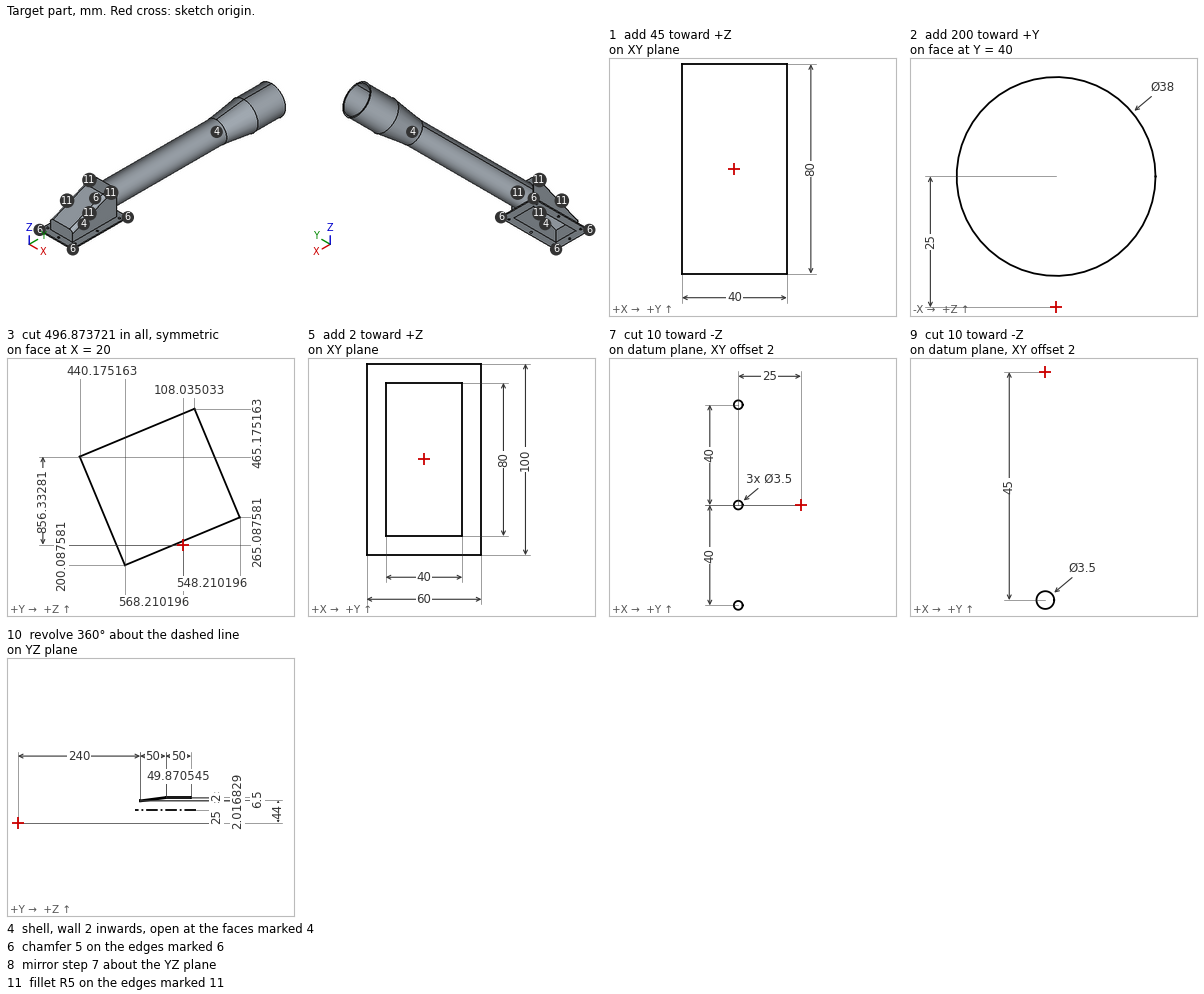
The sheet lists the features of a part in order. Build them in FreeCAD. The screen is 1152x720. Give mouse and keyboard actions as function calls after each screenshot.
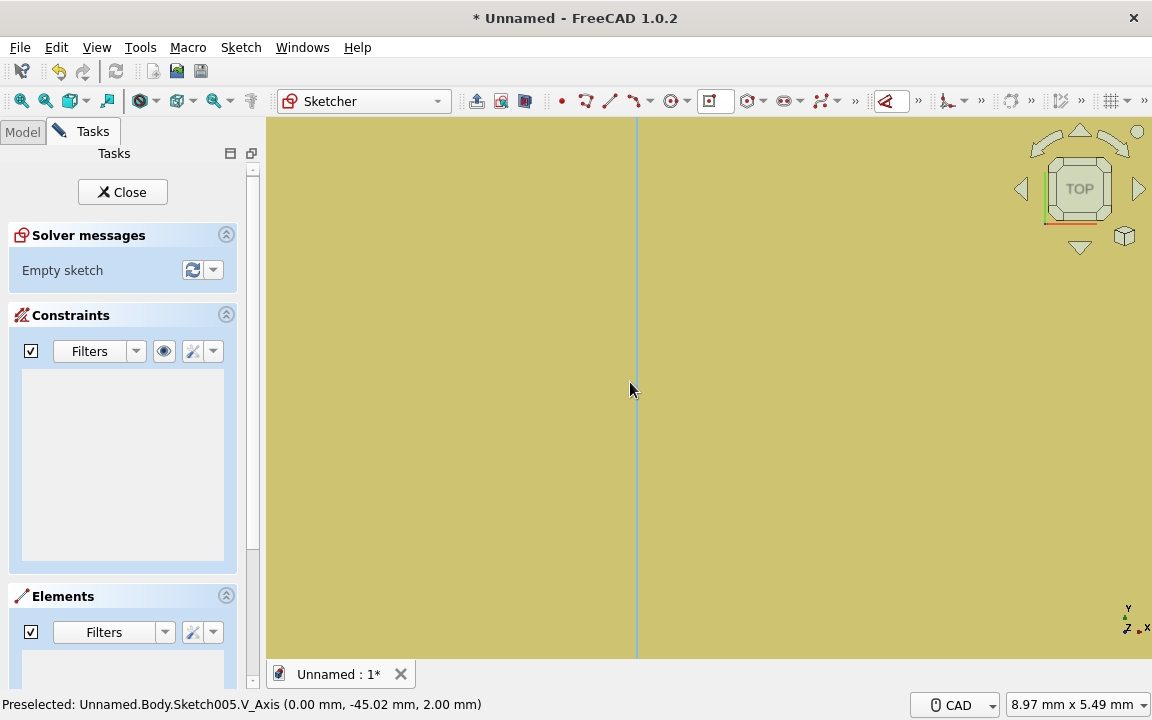
click(672, 102)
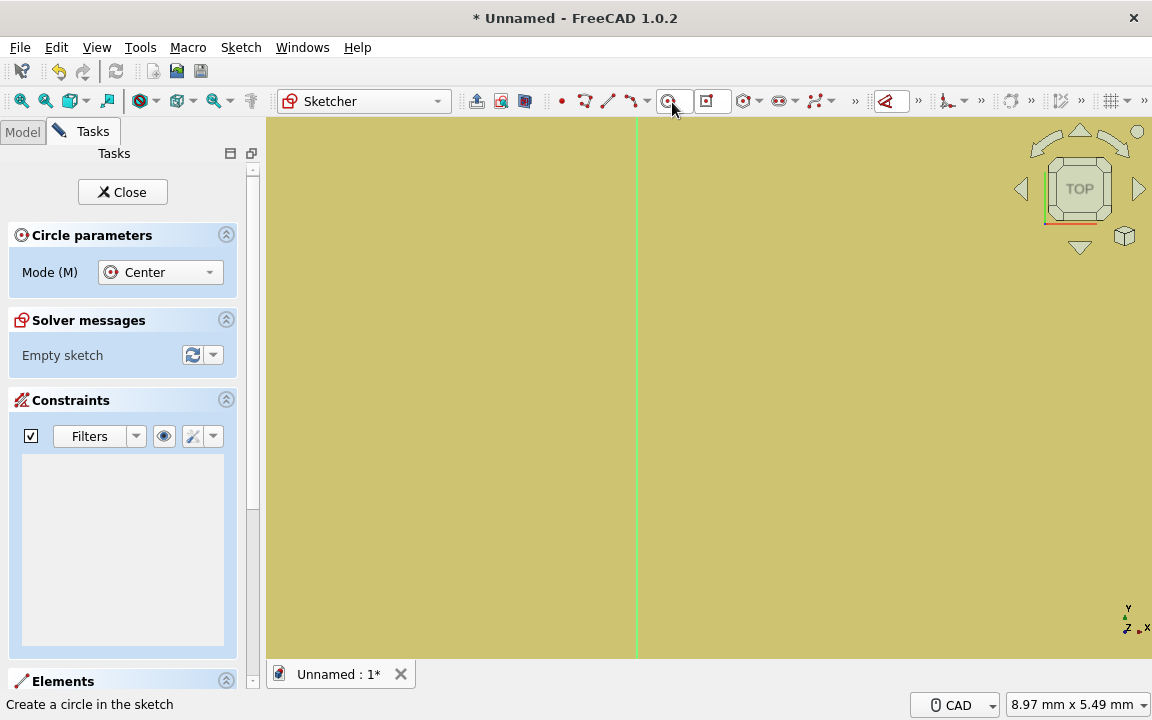
click(637, 384)
move(759, 262)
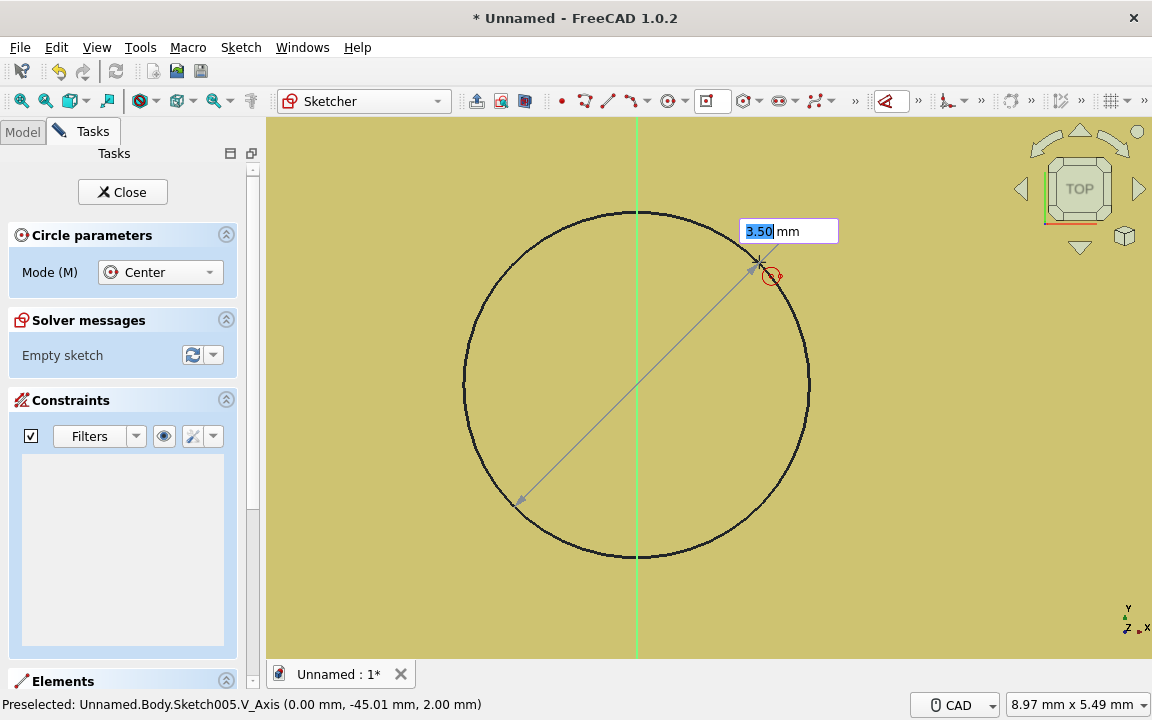
text(3.5)
key(Return)
key(Escape)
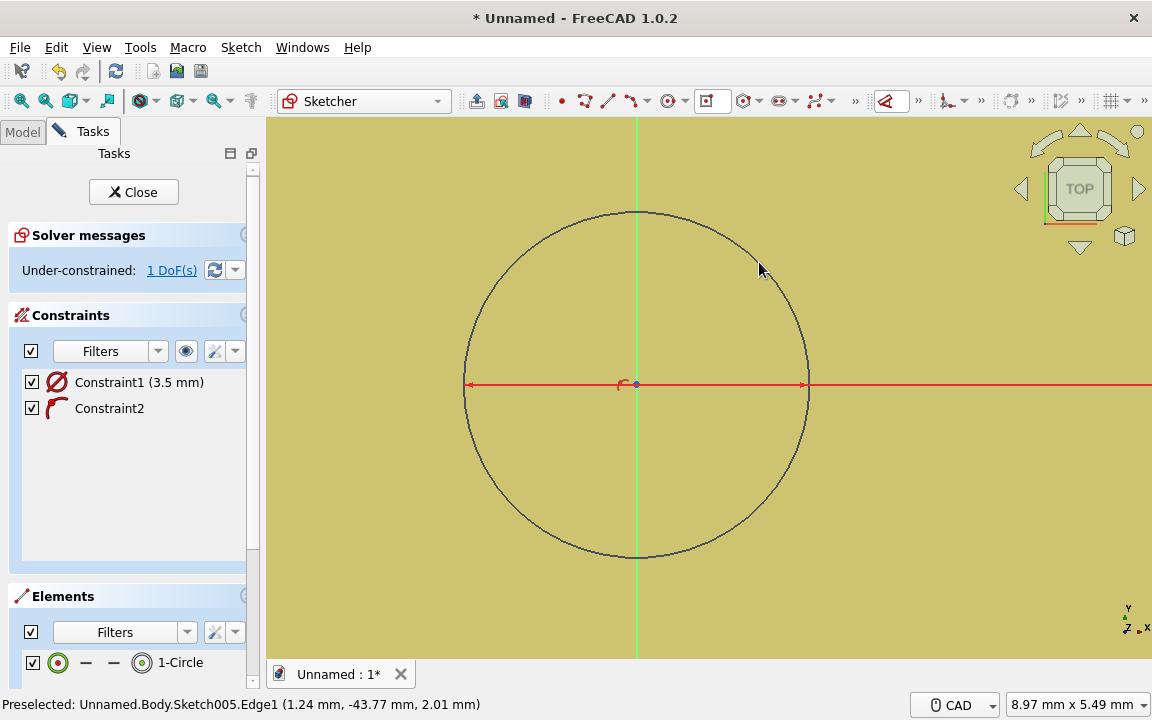
click(886, 102)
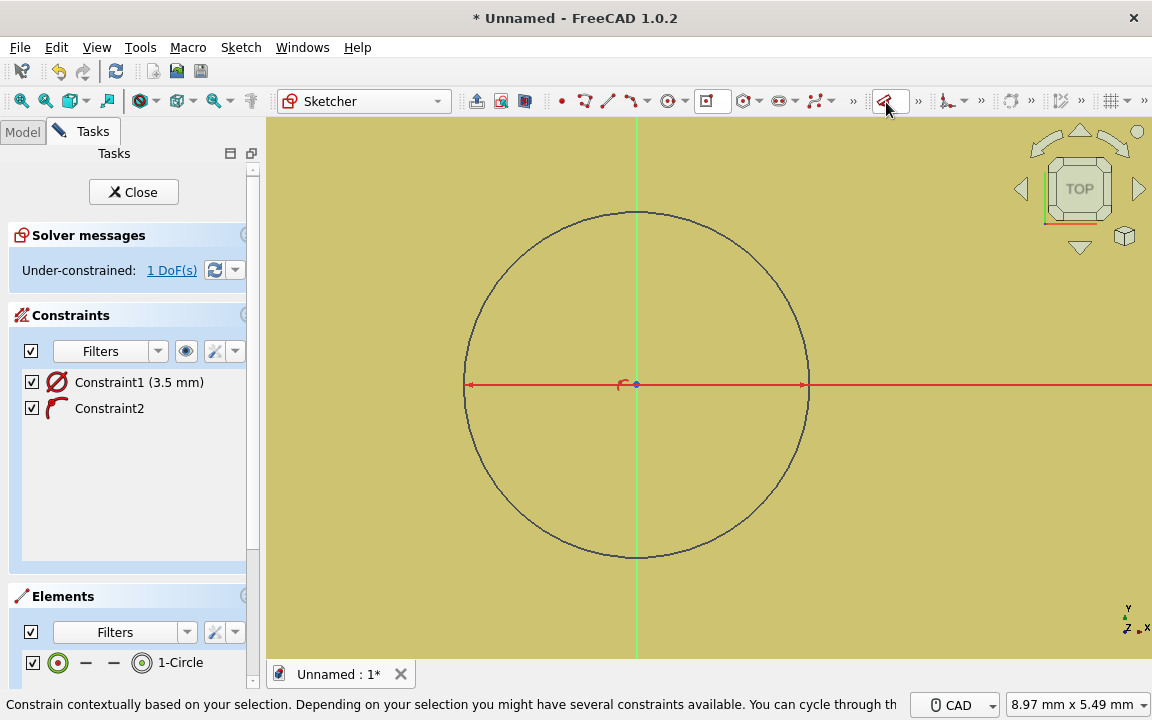
click(637, 385)
click(671, 265)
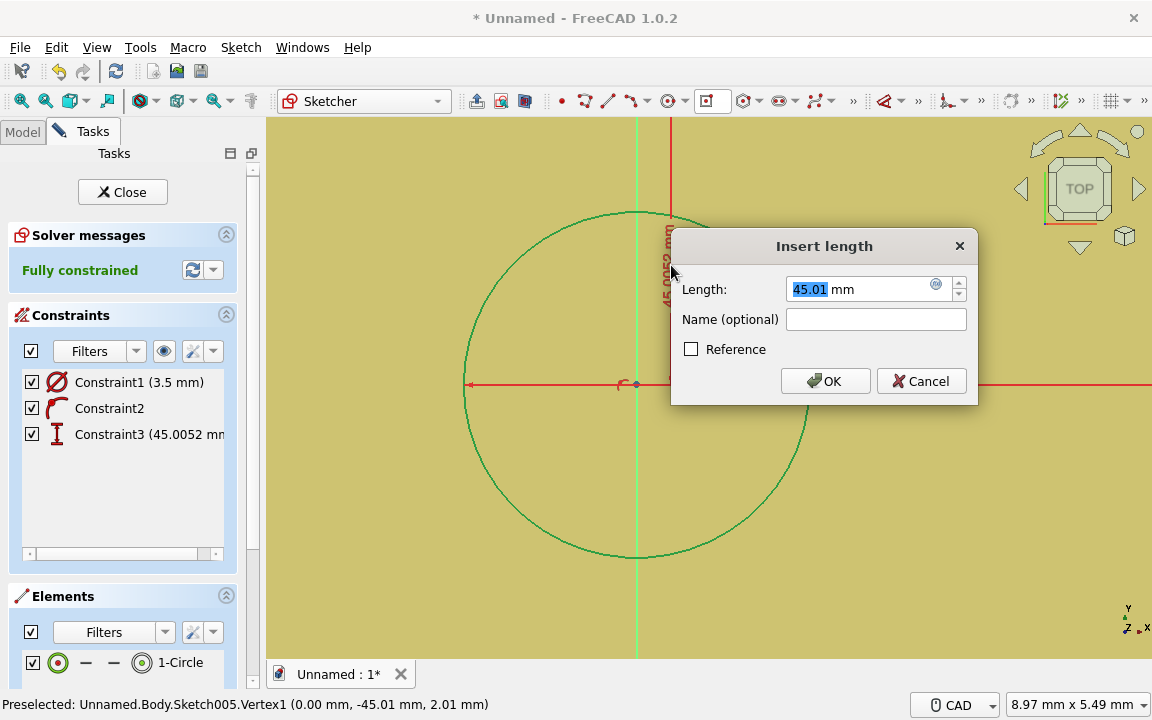
text(45)
key(Return)
key(Escape)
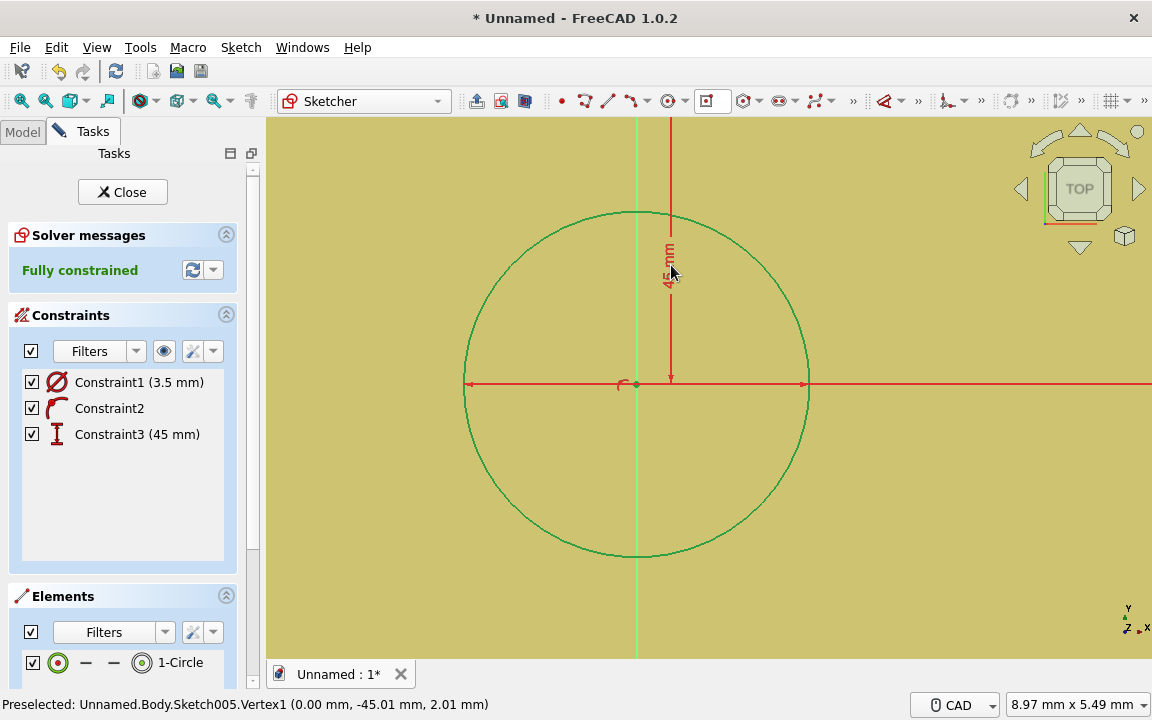
click(123, 192)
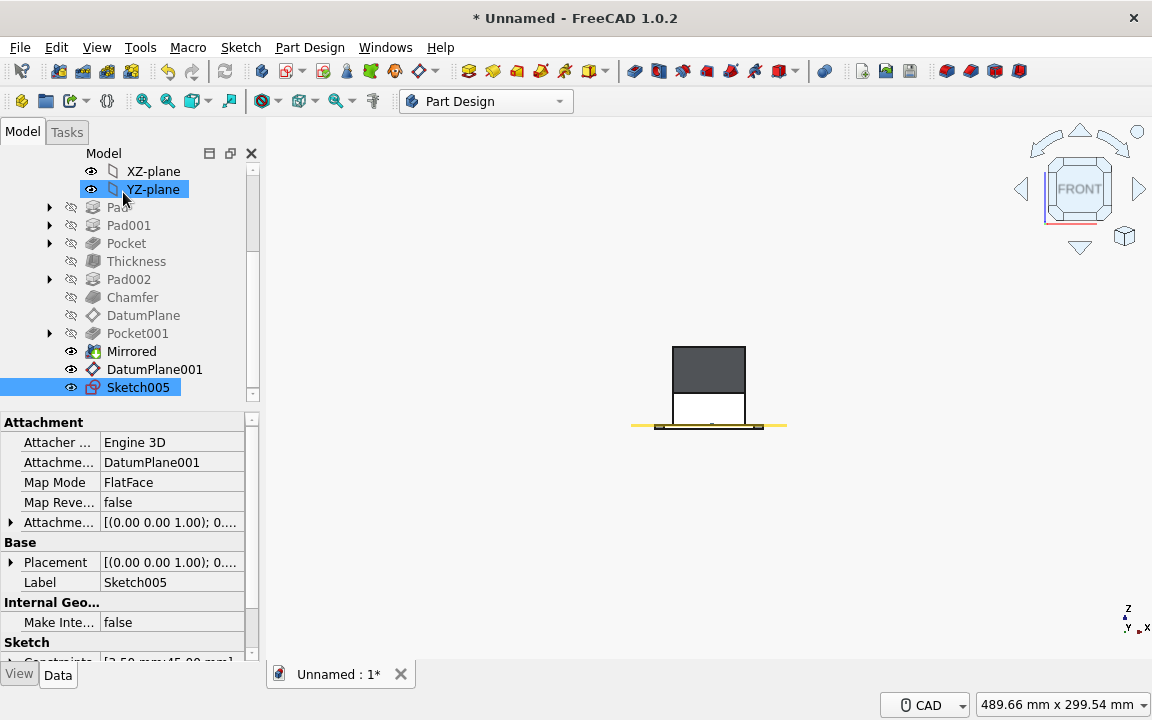
click(636, 72)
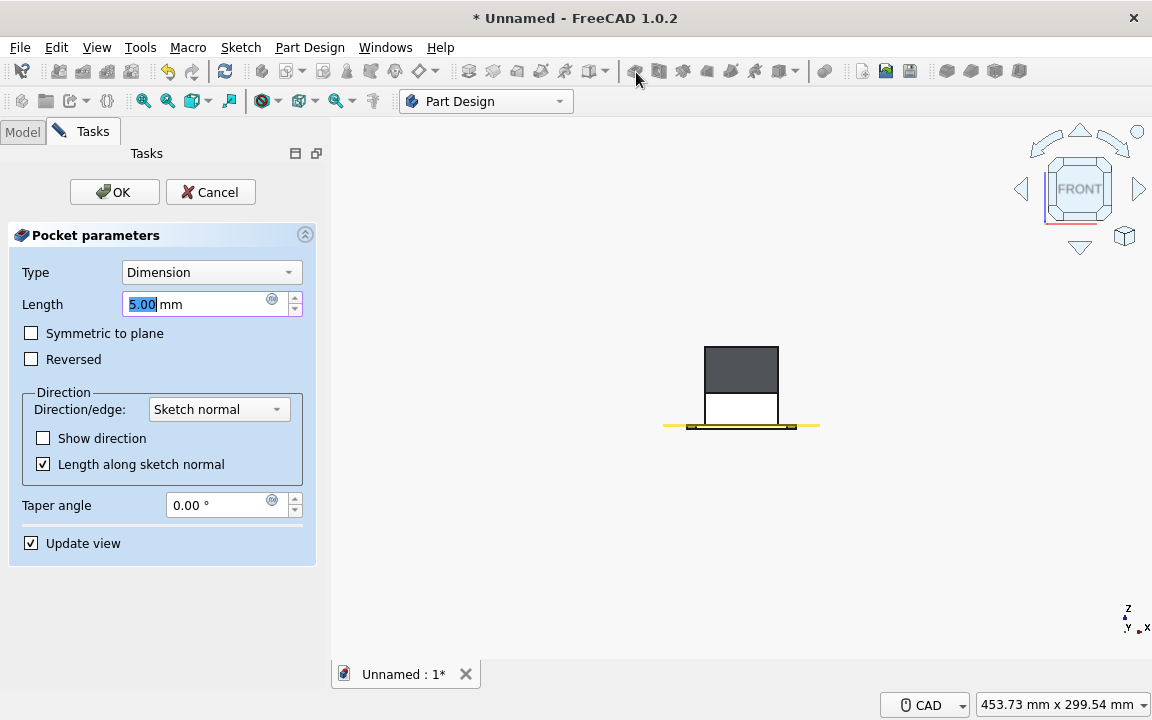
text(10)
key(Tab)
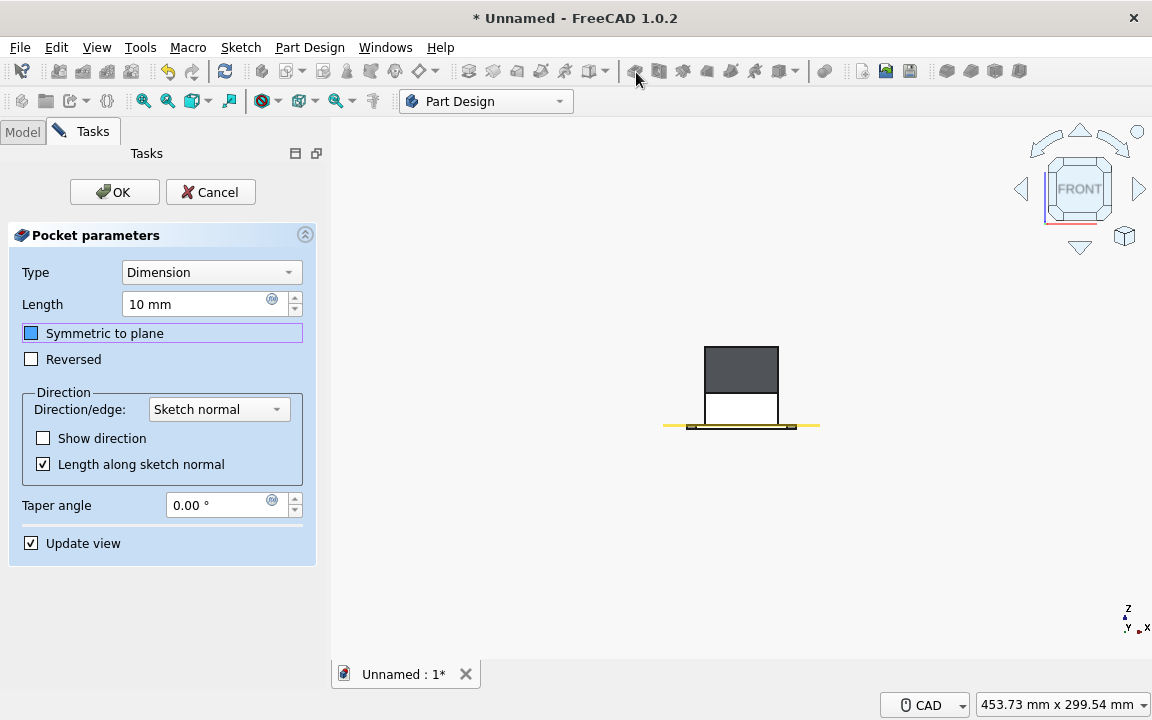
click(115, 192)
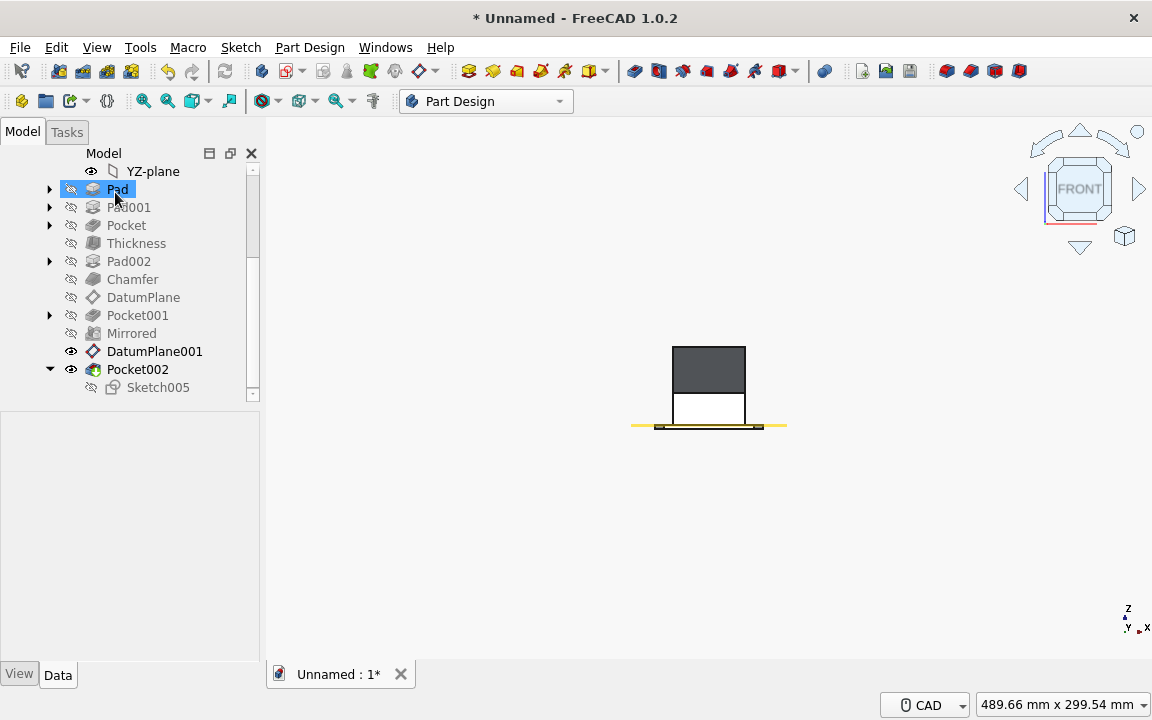
click(116, 351)
key(space)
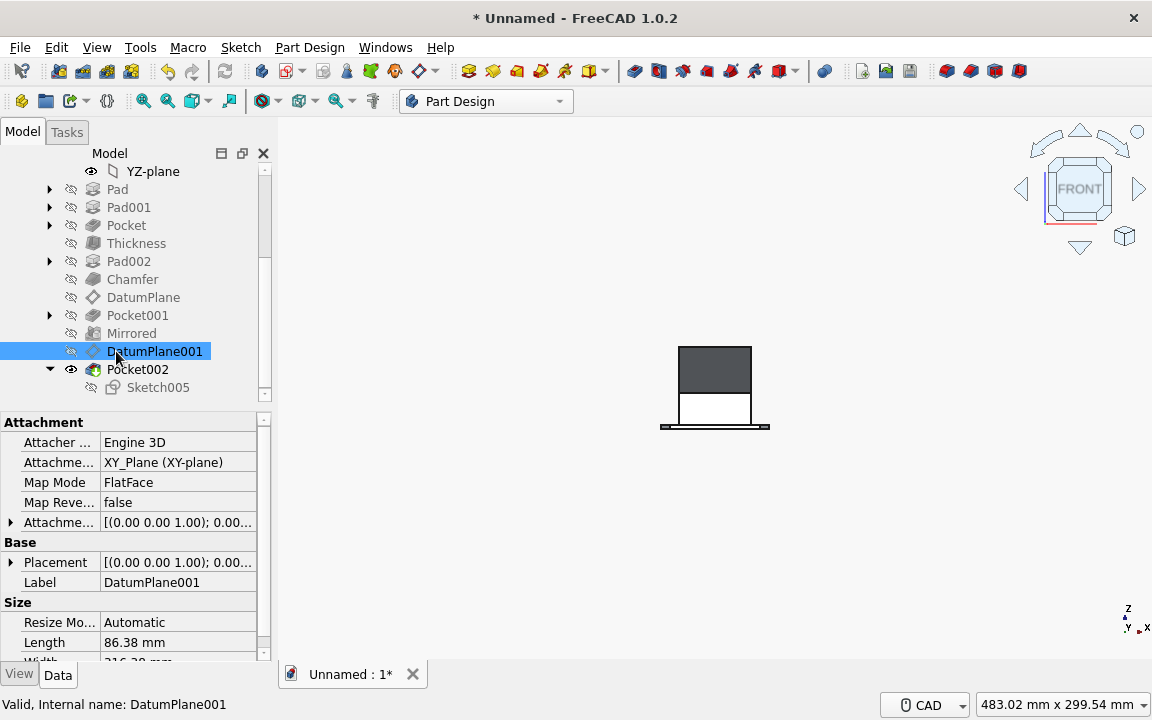
key(v)
key(f)